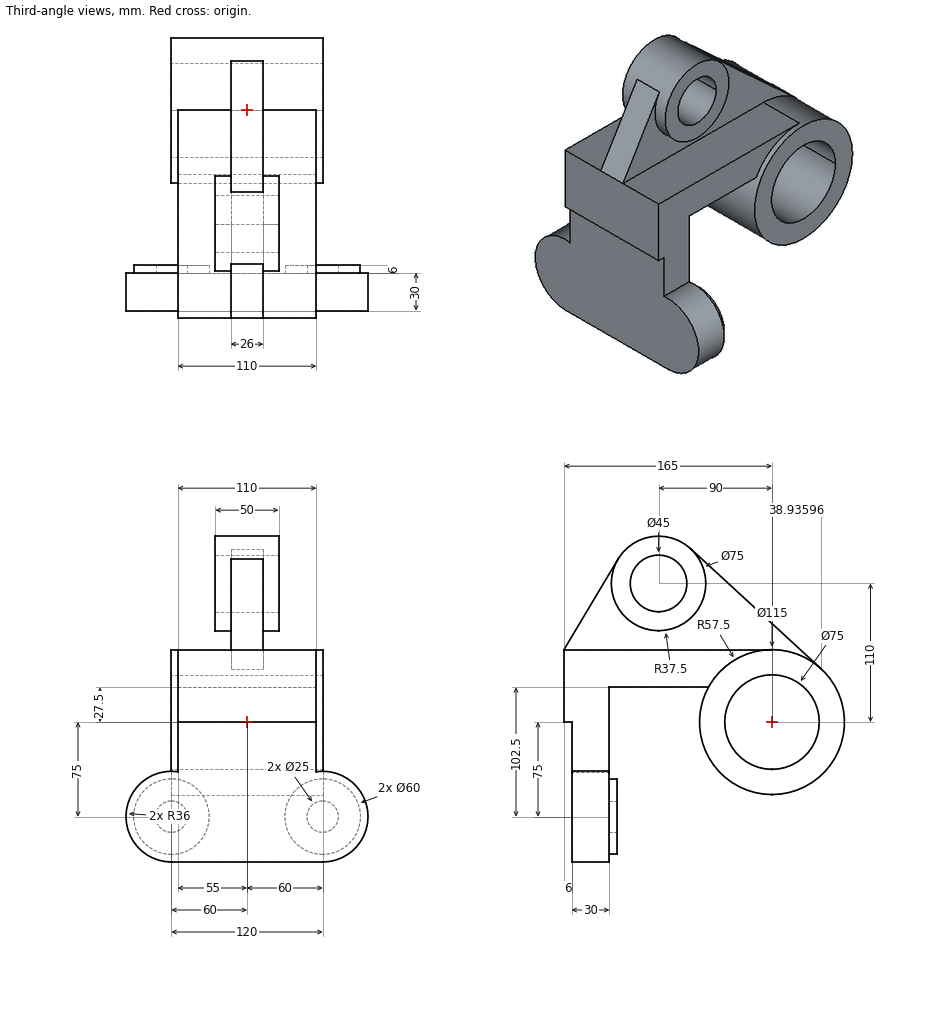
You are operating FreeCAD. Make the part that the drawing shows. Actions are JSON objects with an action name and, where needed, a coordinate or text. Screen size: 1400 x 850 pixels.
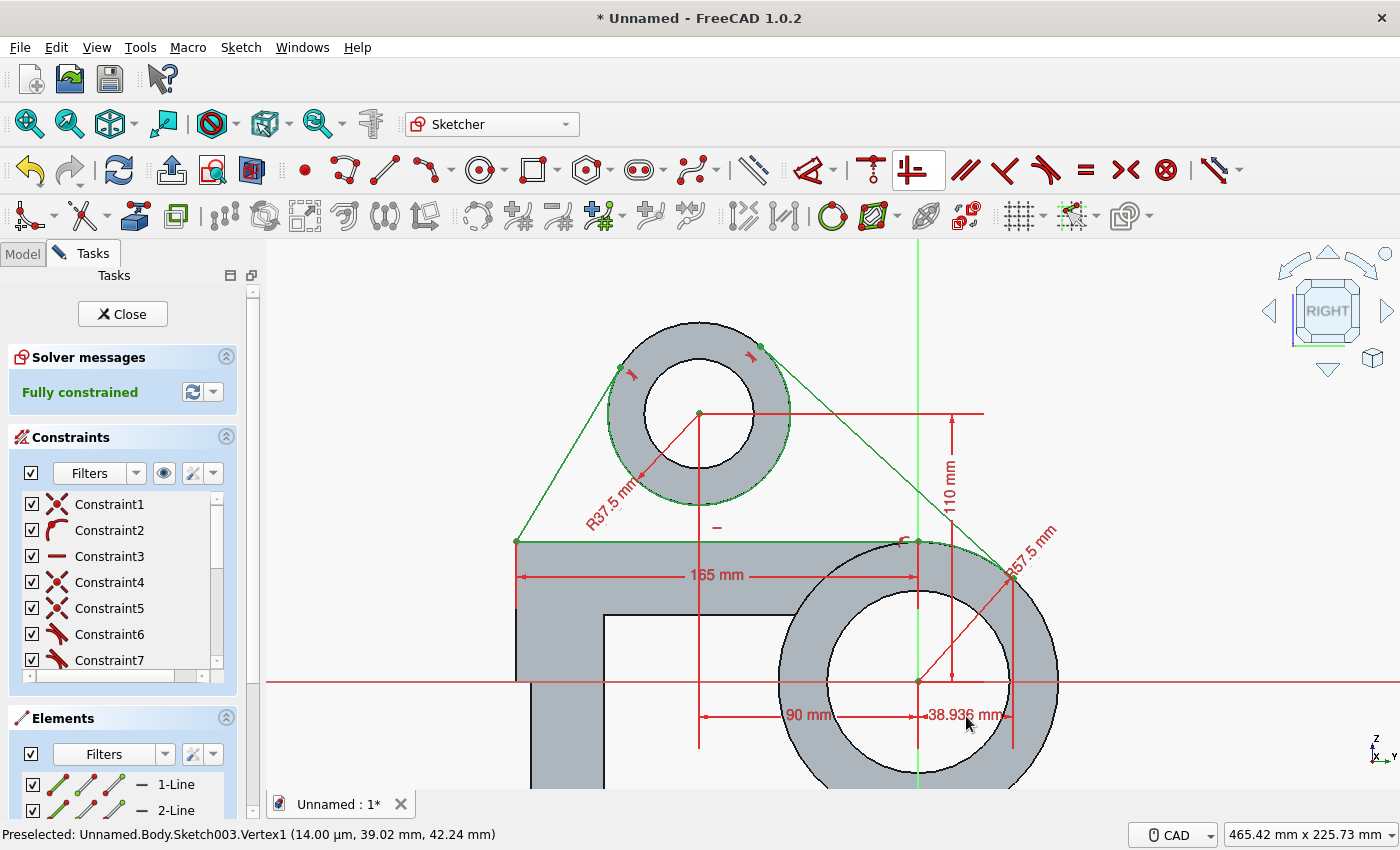
{"action": "left_click", "coordinate": [123, 314]}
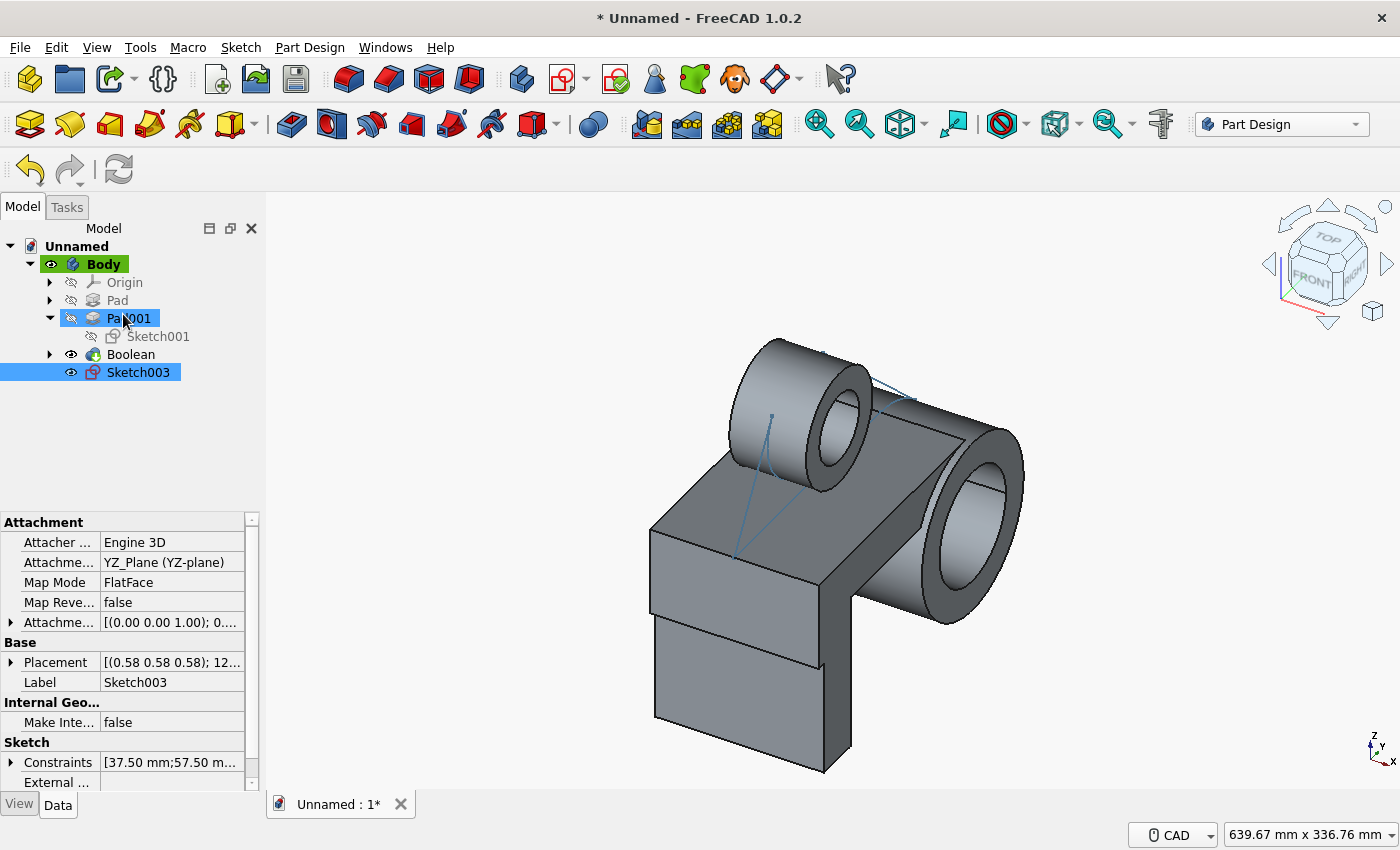
{"action": "left_click", "coordinate": [30, 124]}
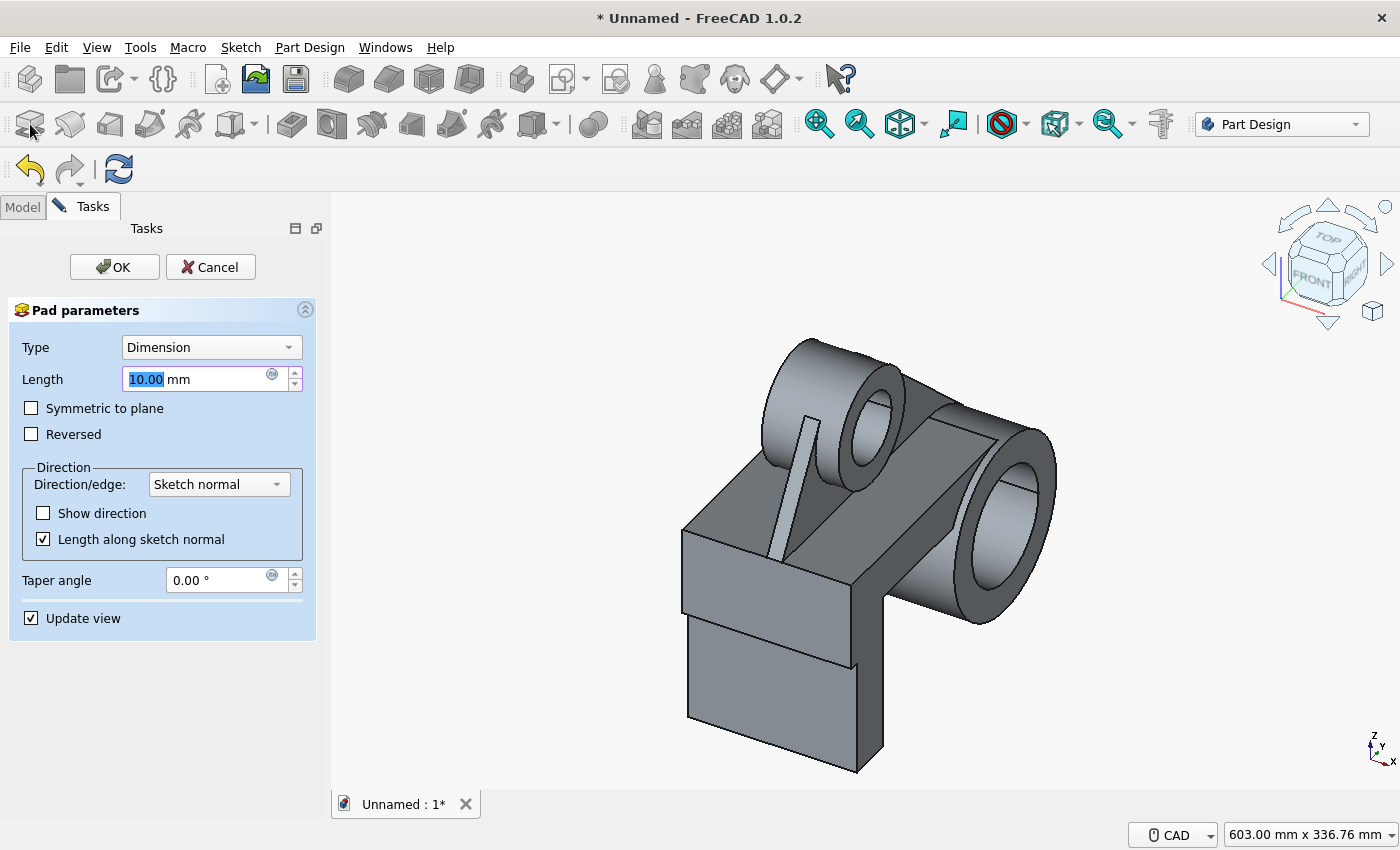
{"action": "type", "text": "26"}
{"action": "key", "text": "Tab"}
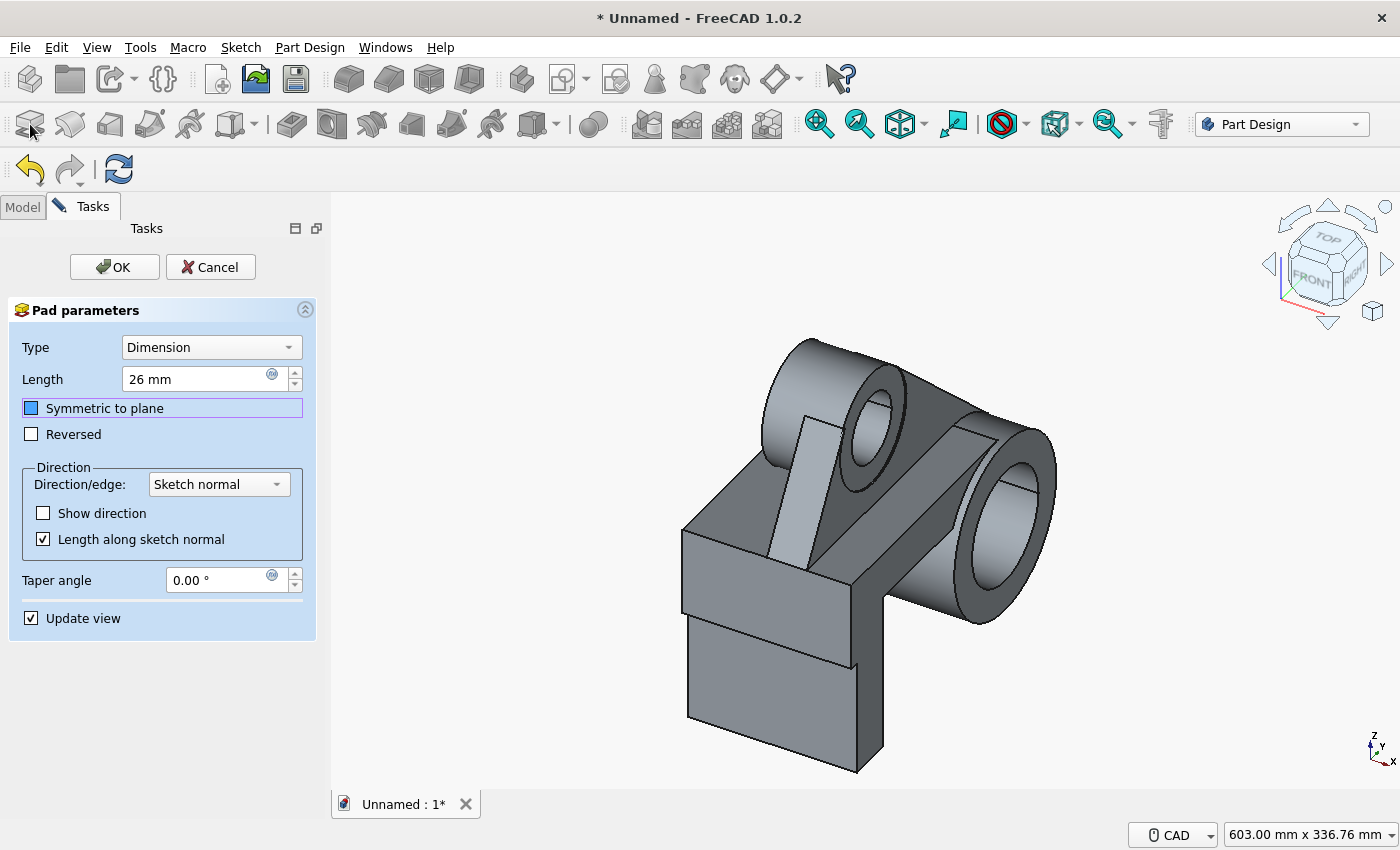
{"action": "left_click", "coordinate": [30, 408]}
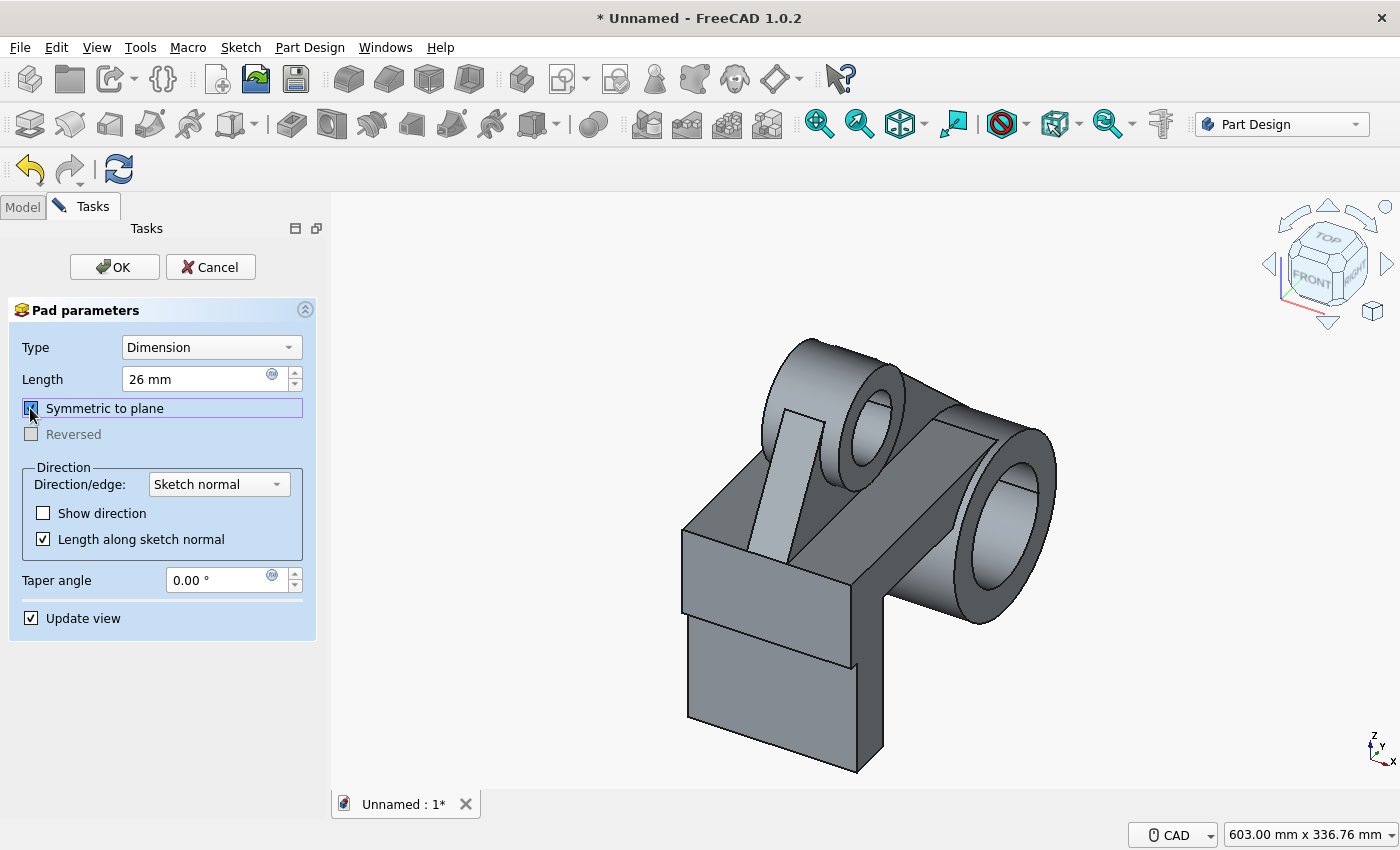
{"action": "left_click", "coordinate": [115, 267]}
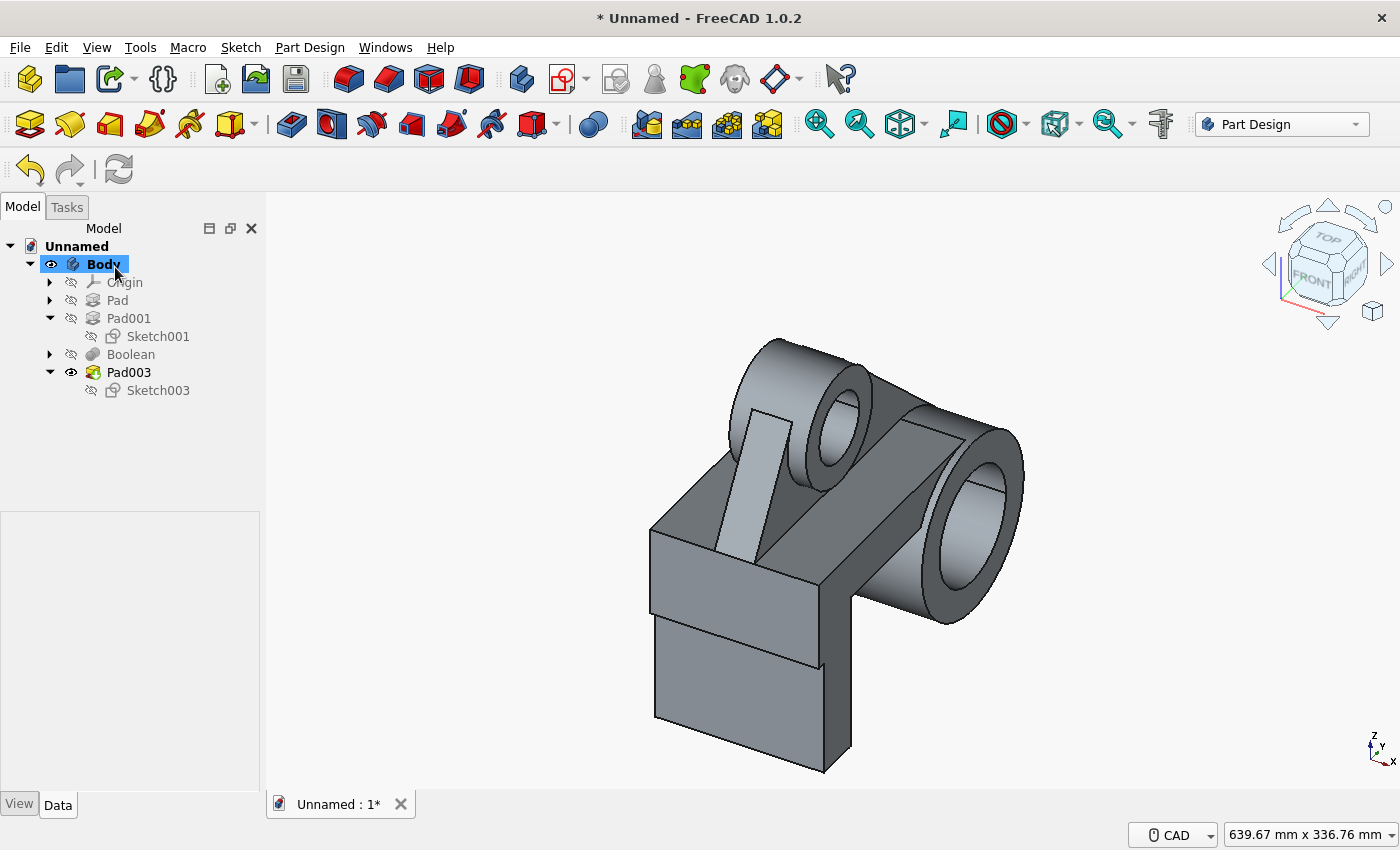
{"action": "left_click", "coordinate": [50, 282]}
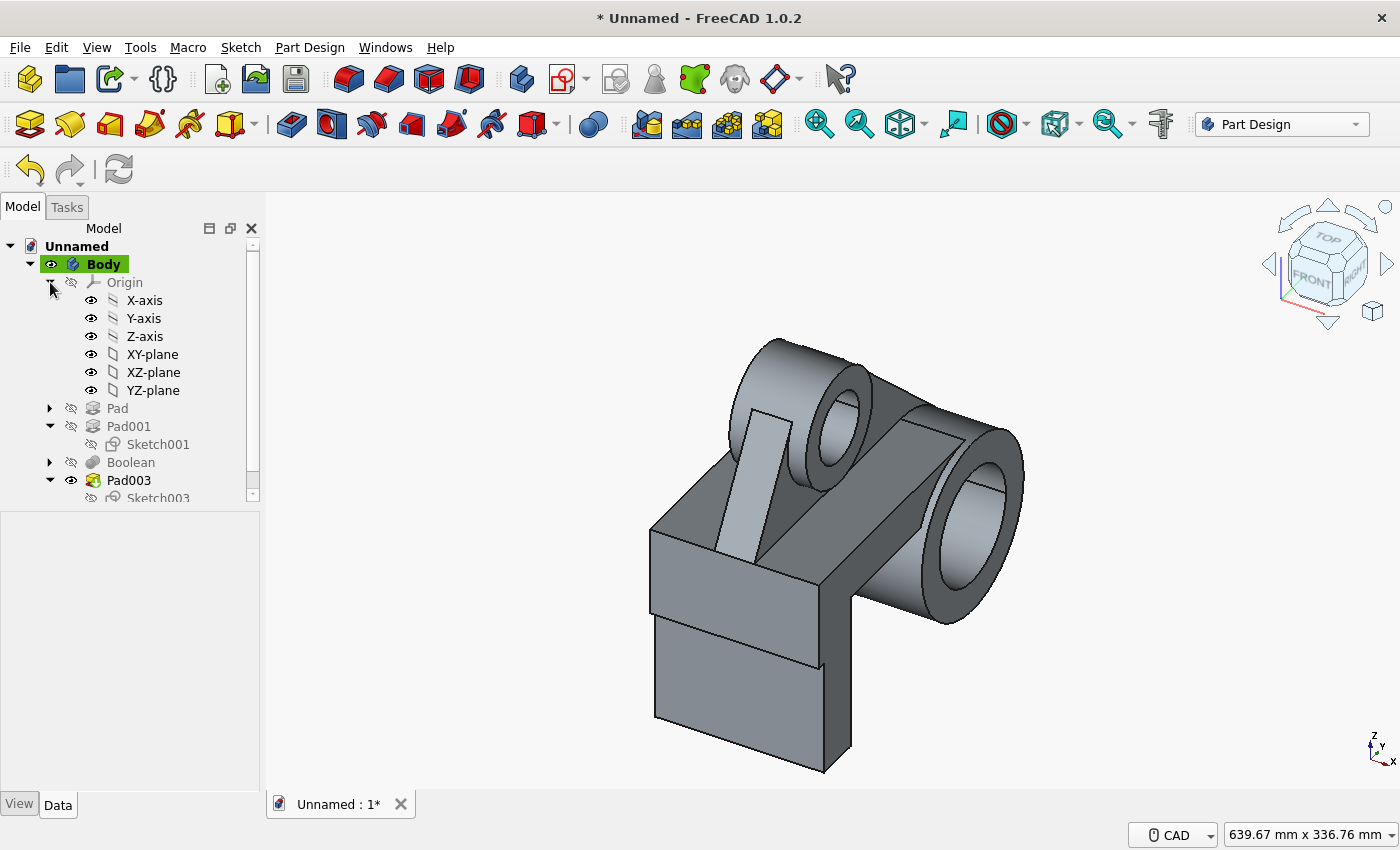
{"action": "left_click", "coordinate": [136, 372]}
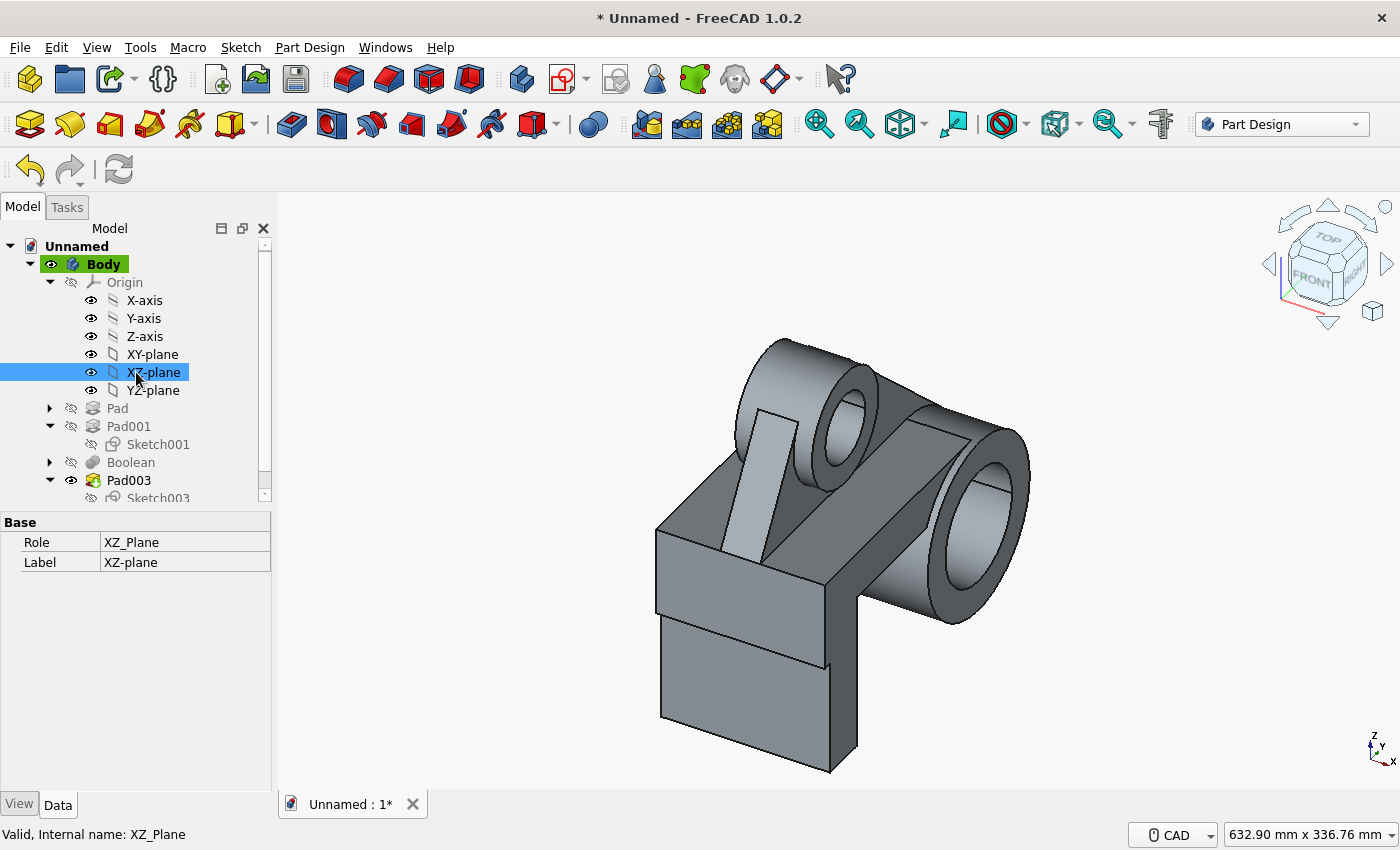
{"action": "left_click", "coordinate": [776, 80]}